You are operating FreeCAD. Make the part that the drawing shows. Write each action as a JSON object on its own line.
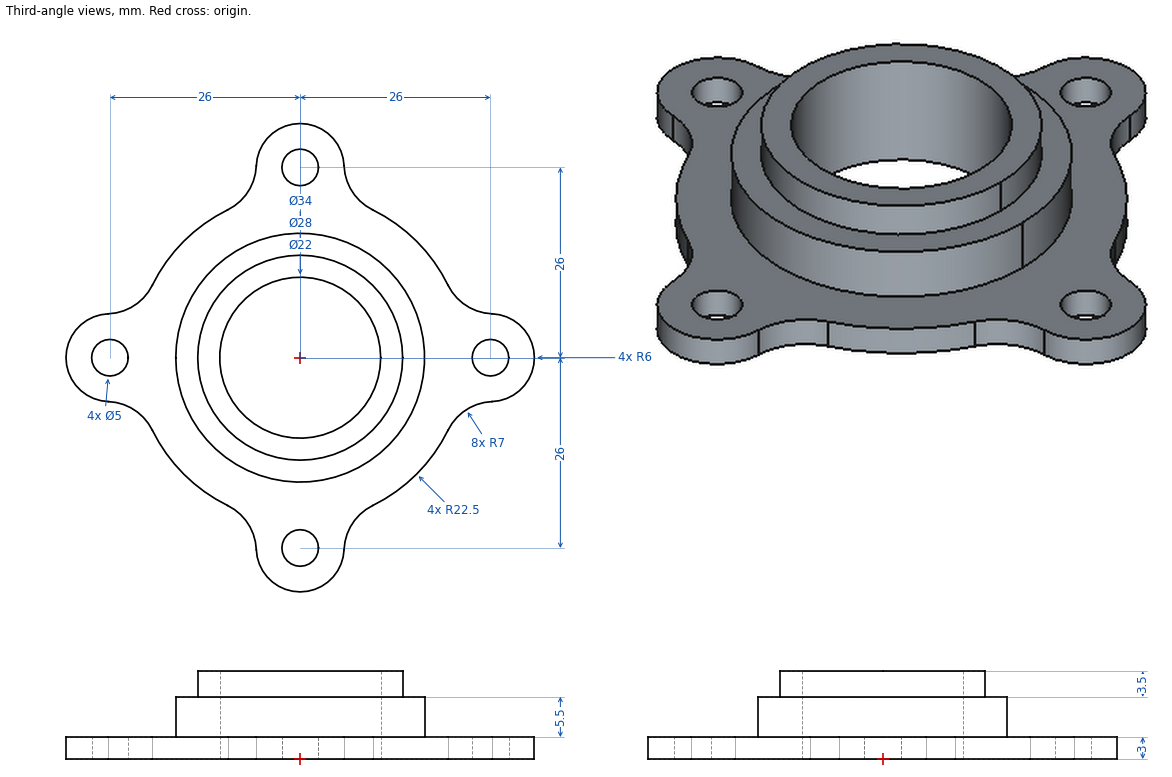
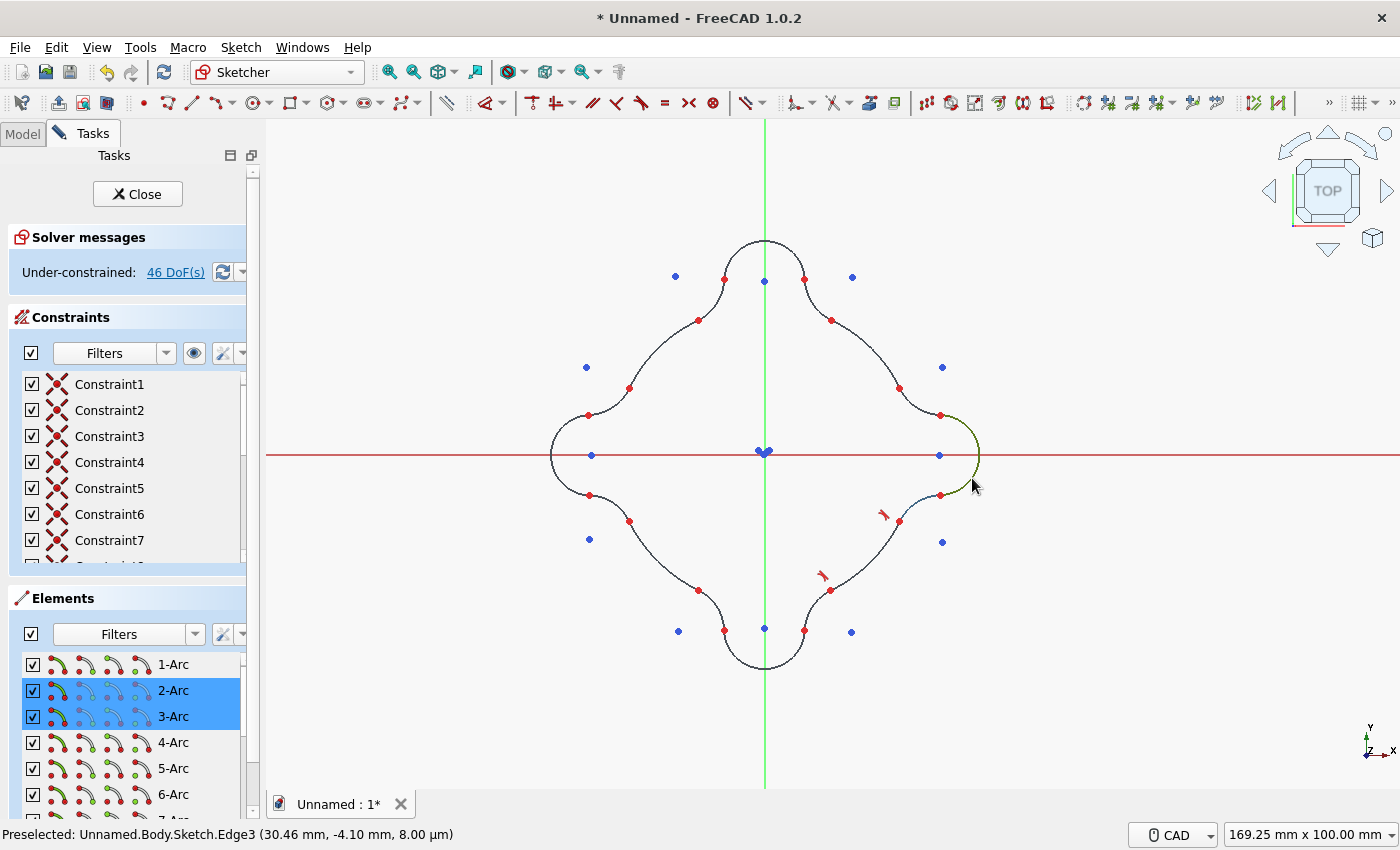
{"action": "left_click", "coordinate": [642, 104]}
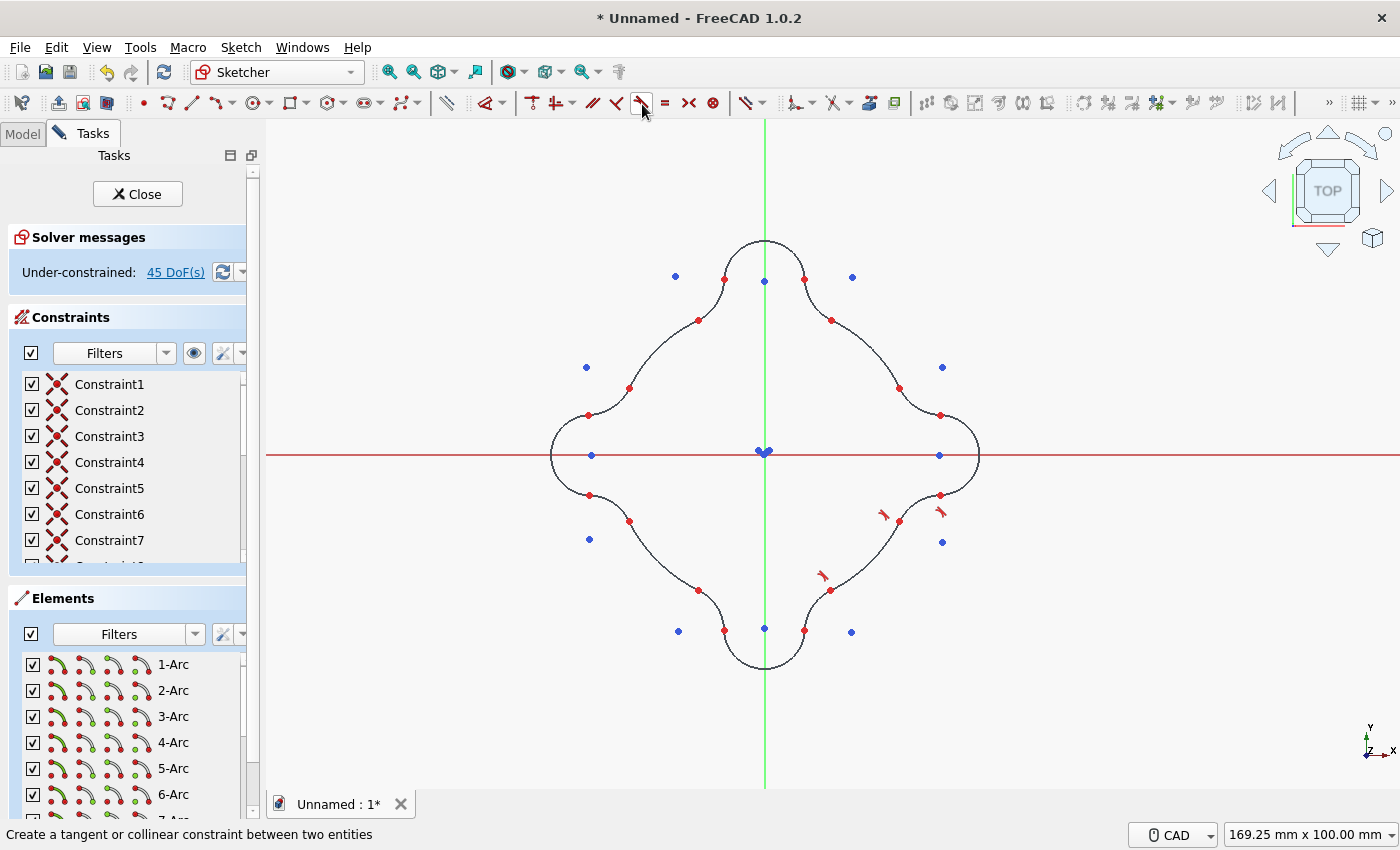
{"action": "left_click", "coordinate": [972, 478]}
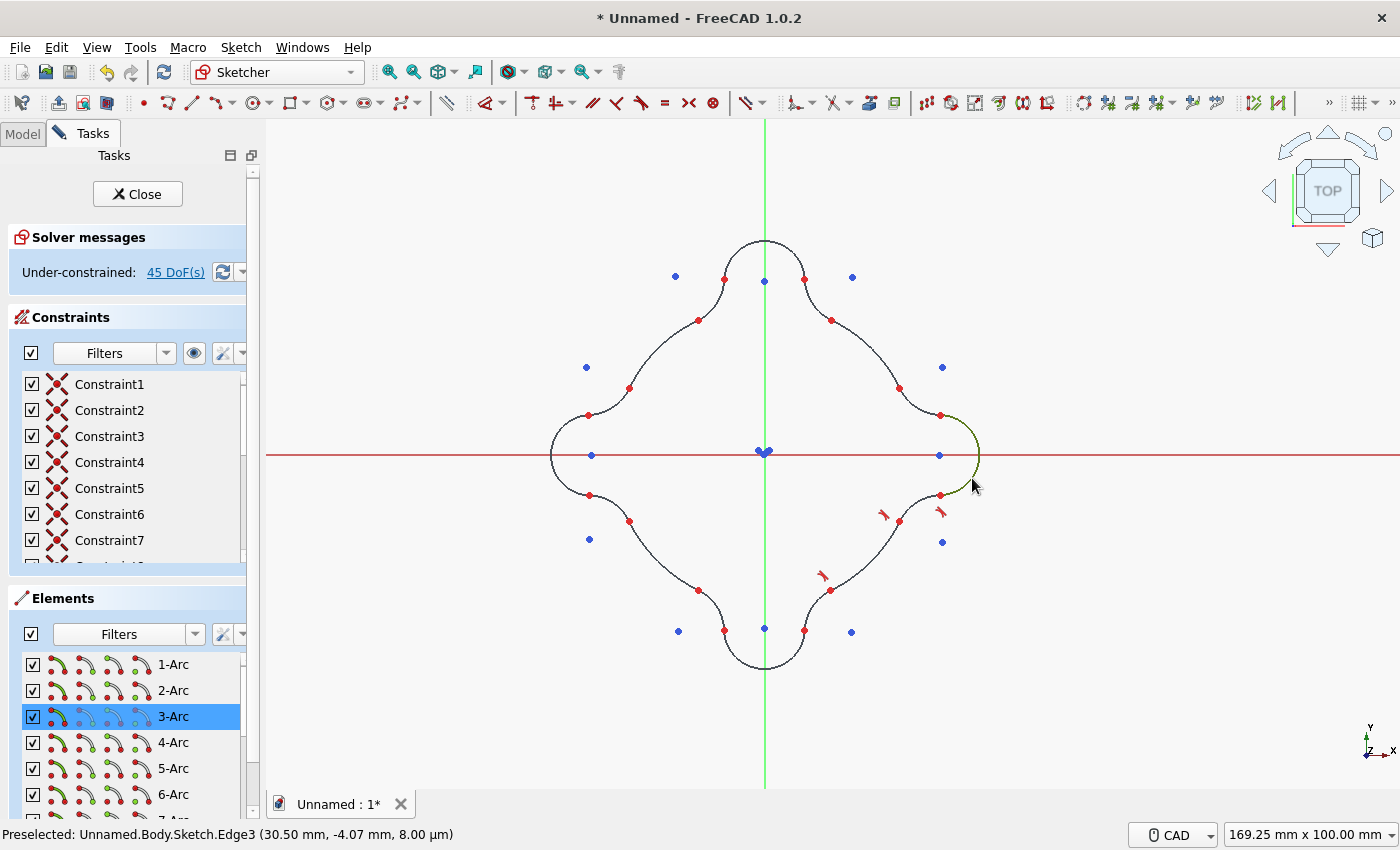
{"action": "left_click", "coordinate": [909, 401]}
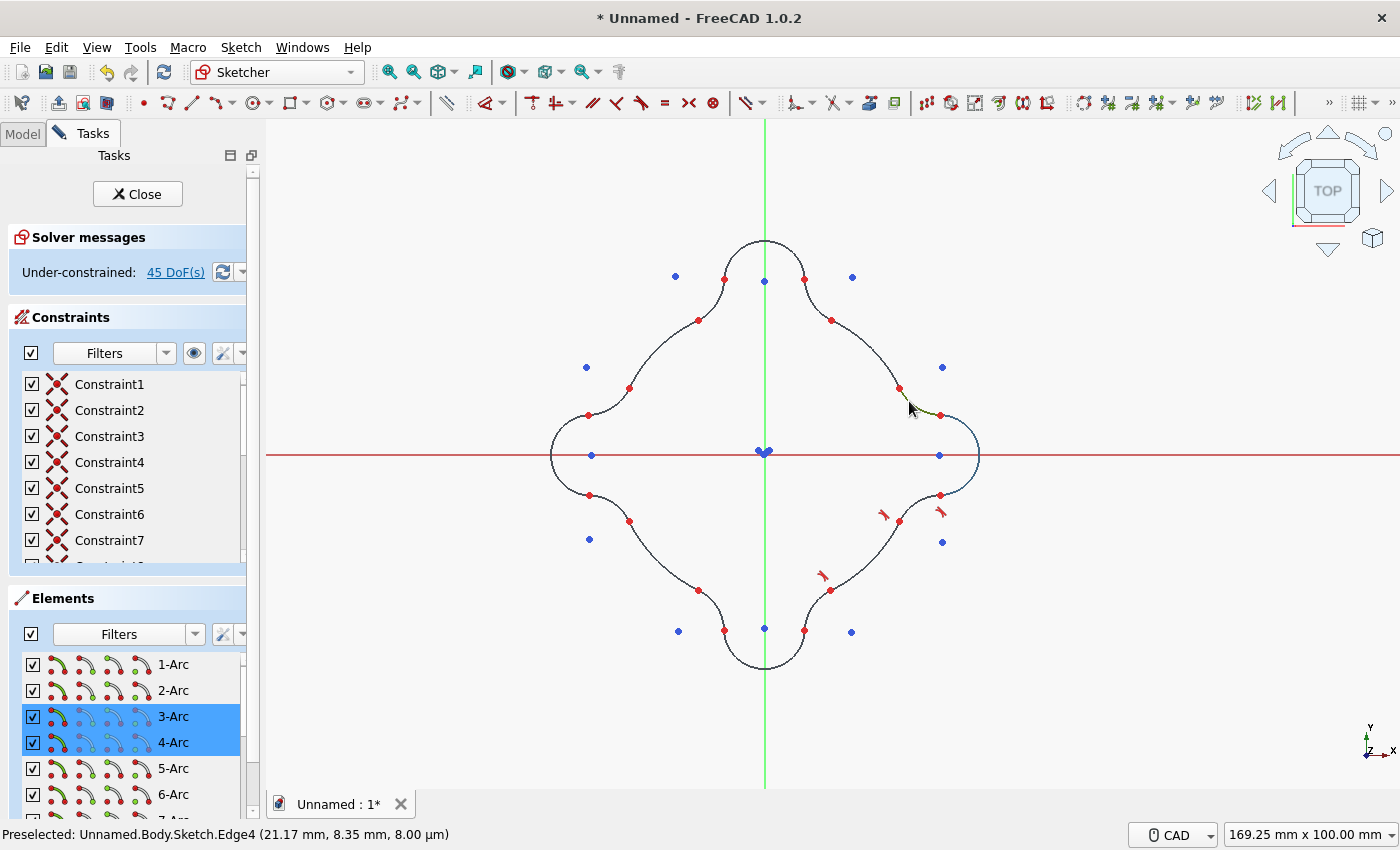
{"action": "left_click", "coordinate": [642, 104]}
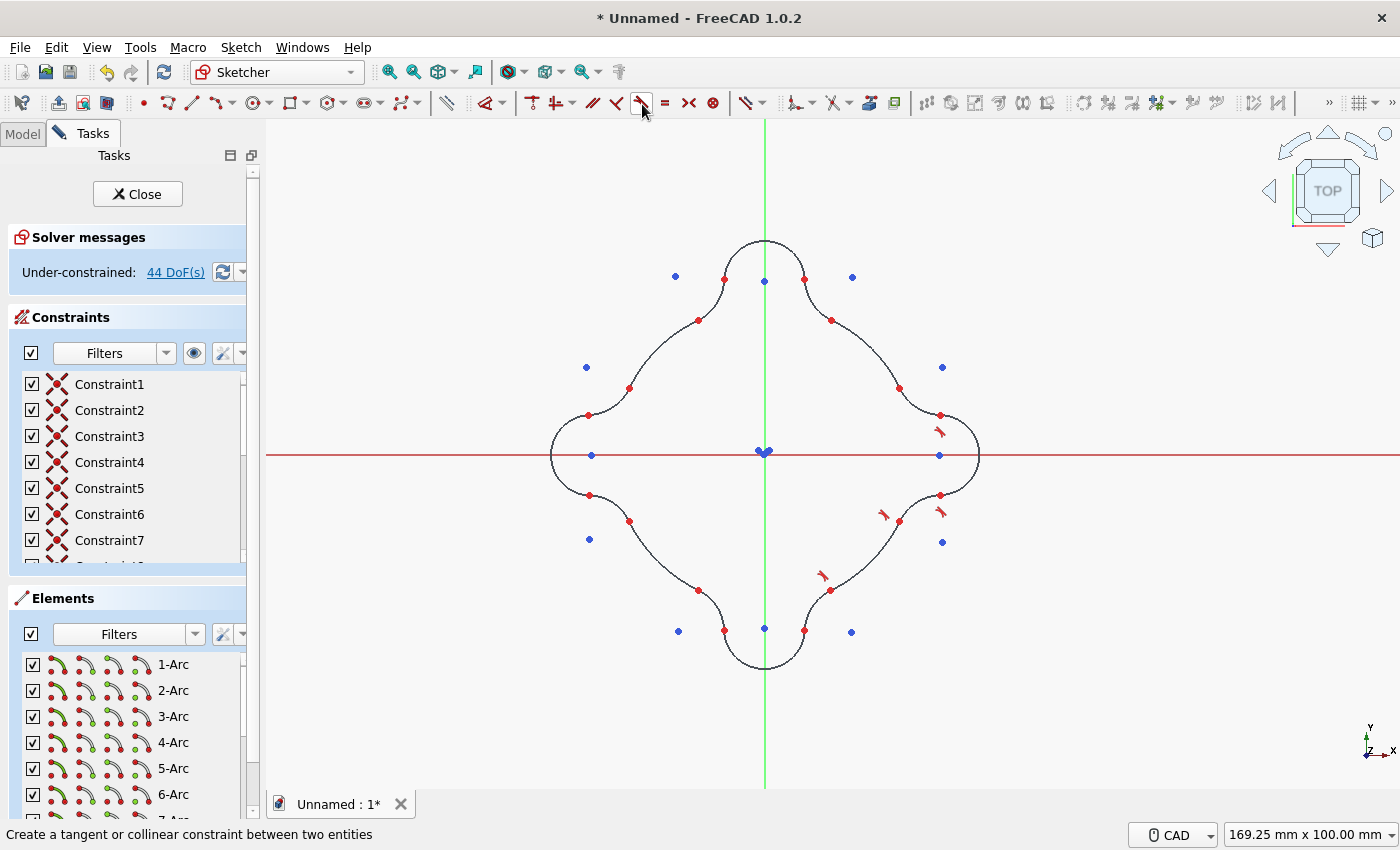
{"action": "left_click", "coordinate": [909, 401]}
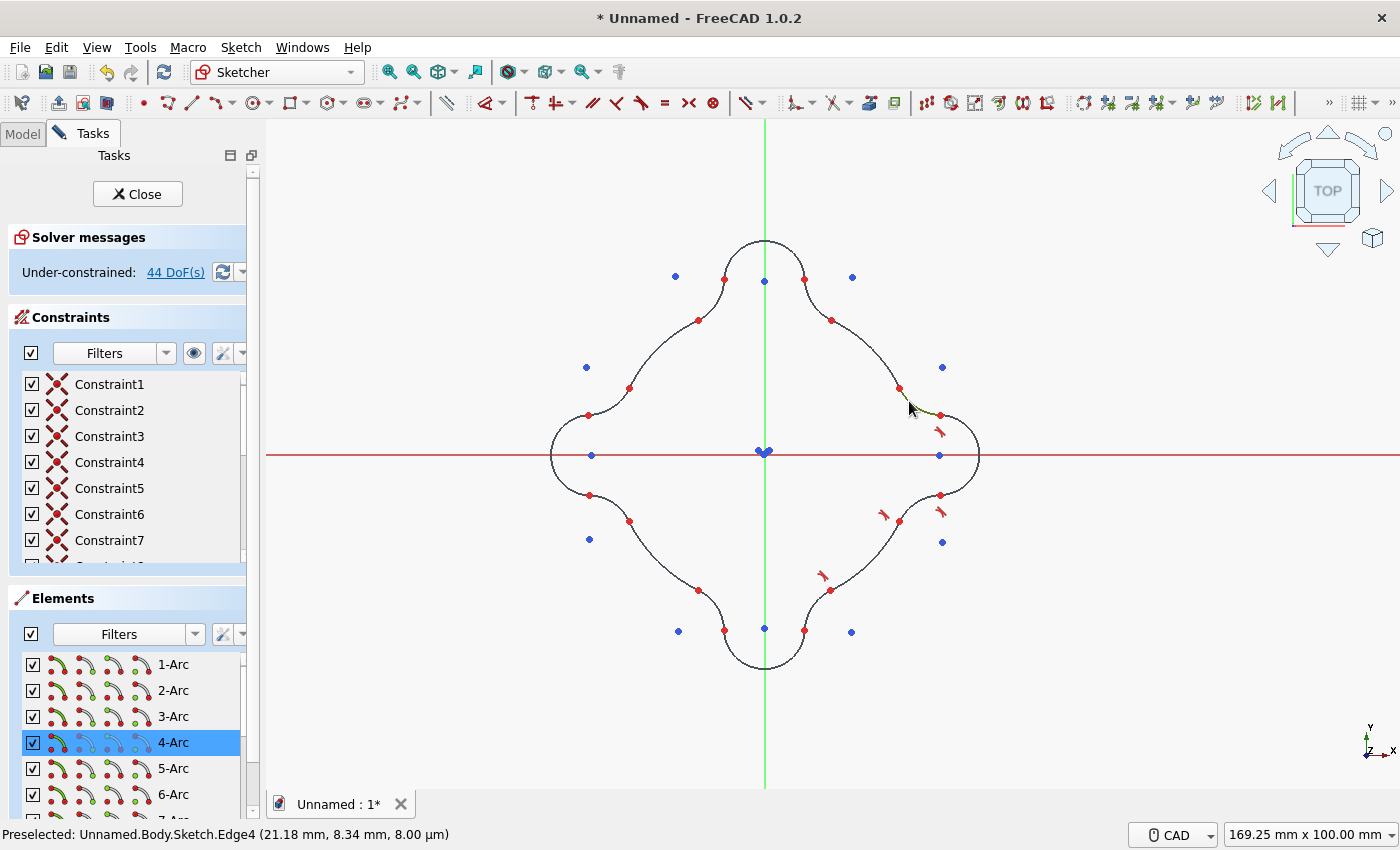
{"action": "left_click", "coordinate": [884, 363]}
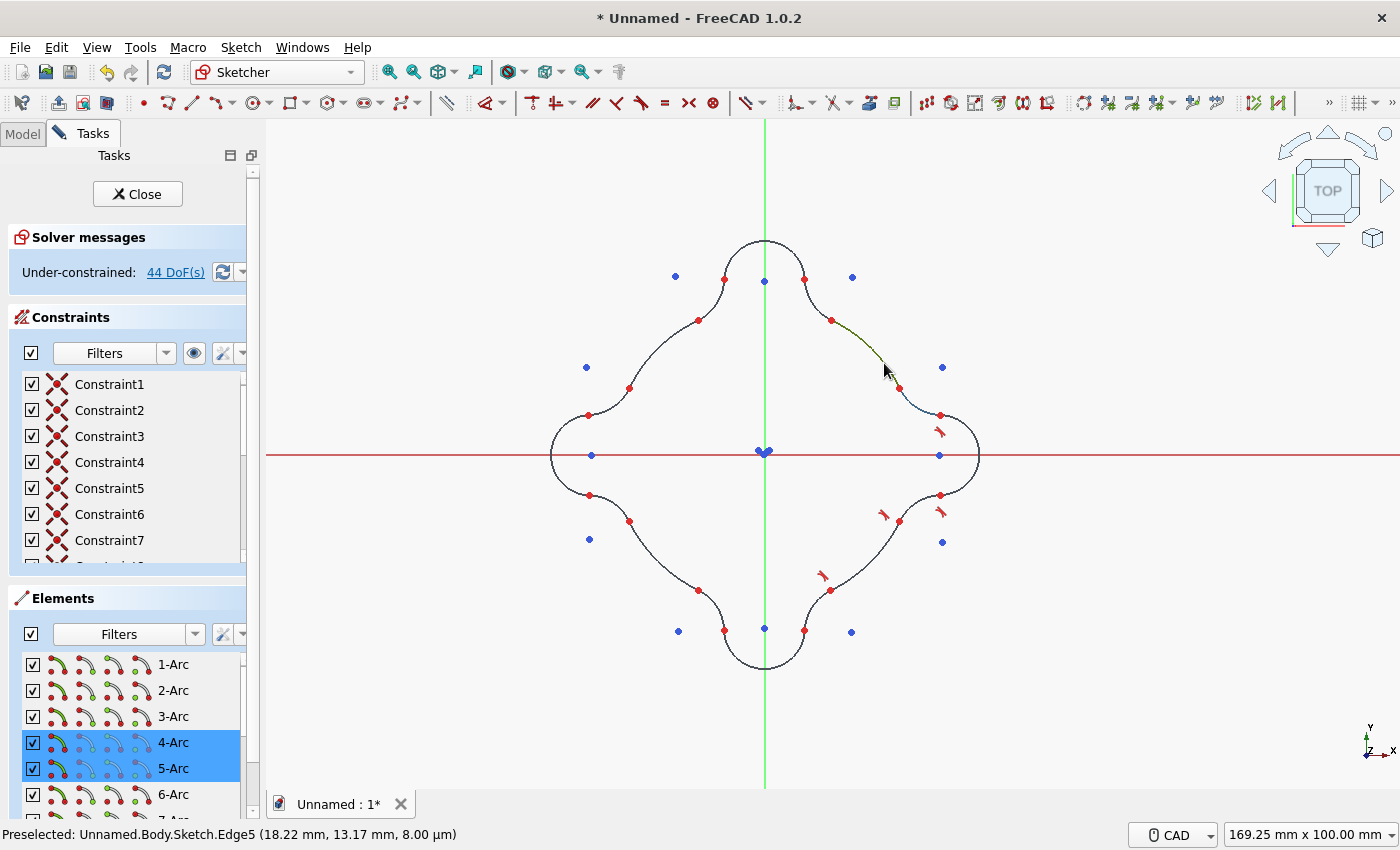
{"action": "left_click", "coordinate": [642, 104]}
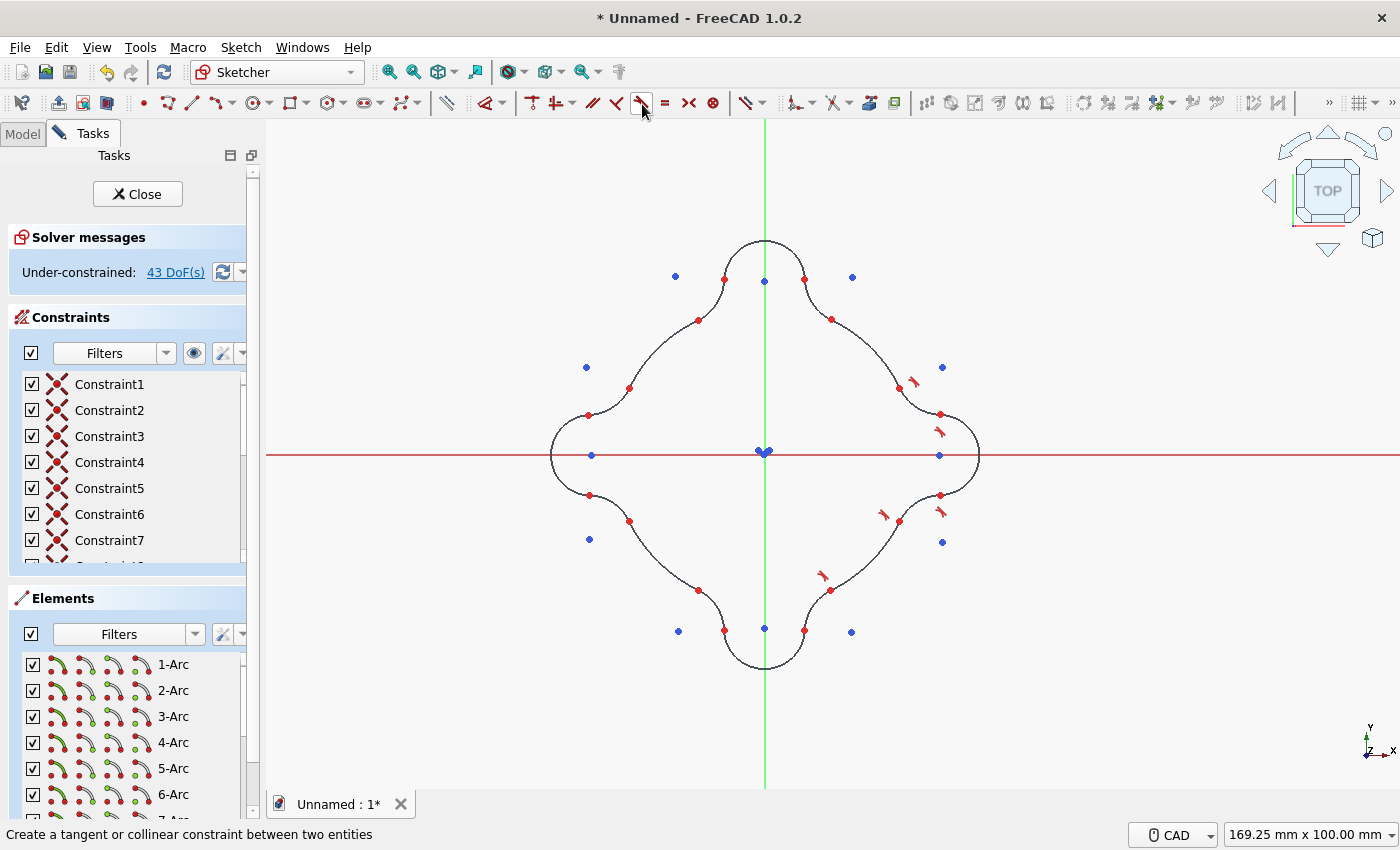
{"action": "left_click", "coordinate": [884, 363]}